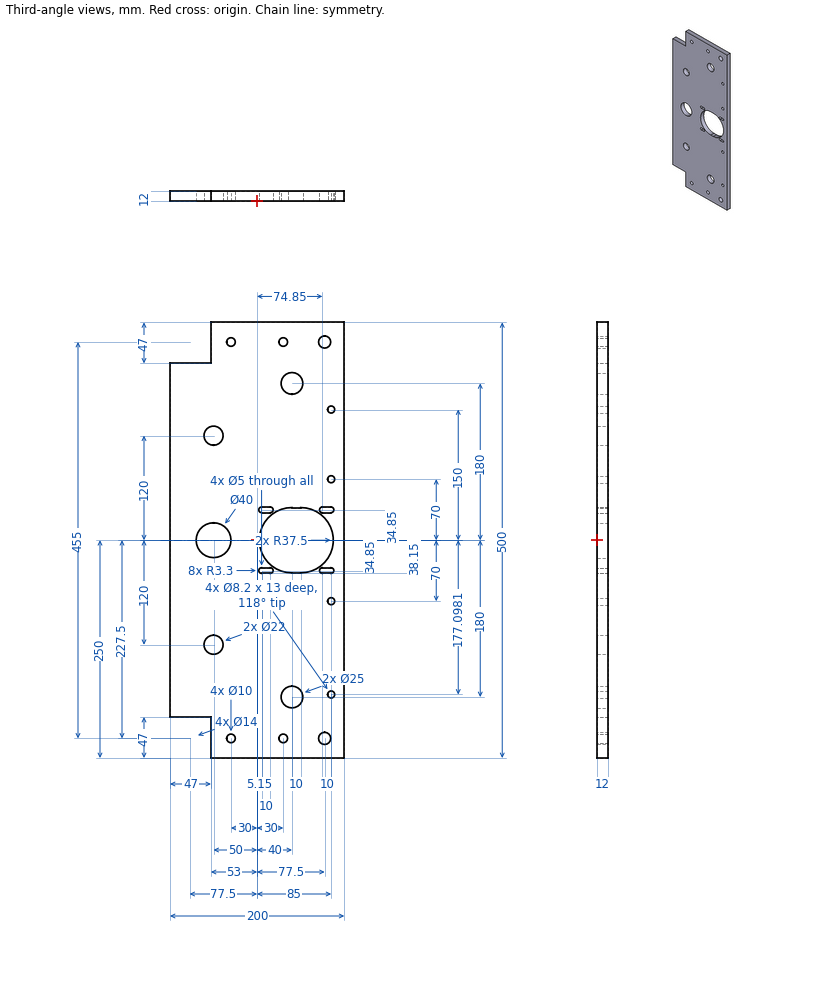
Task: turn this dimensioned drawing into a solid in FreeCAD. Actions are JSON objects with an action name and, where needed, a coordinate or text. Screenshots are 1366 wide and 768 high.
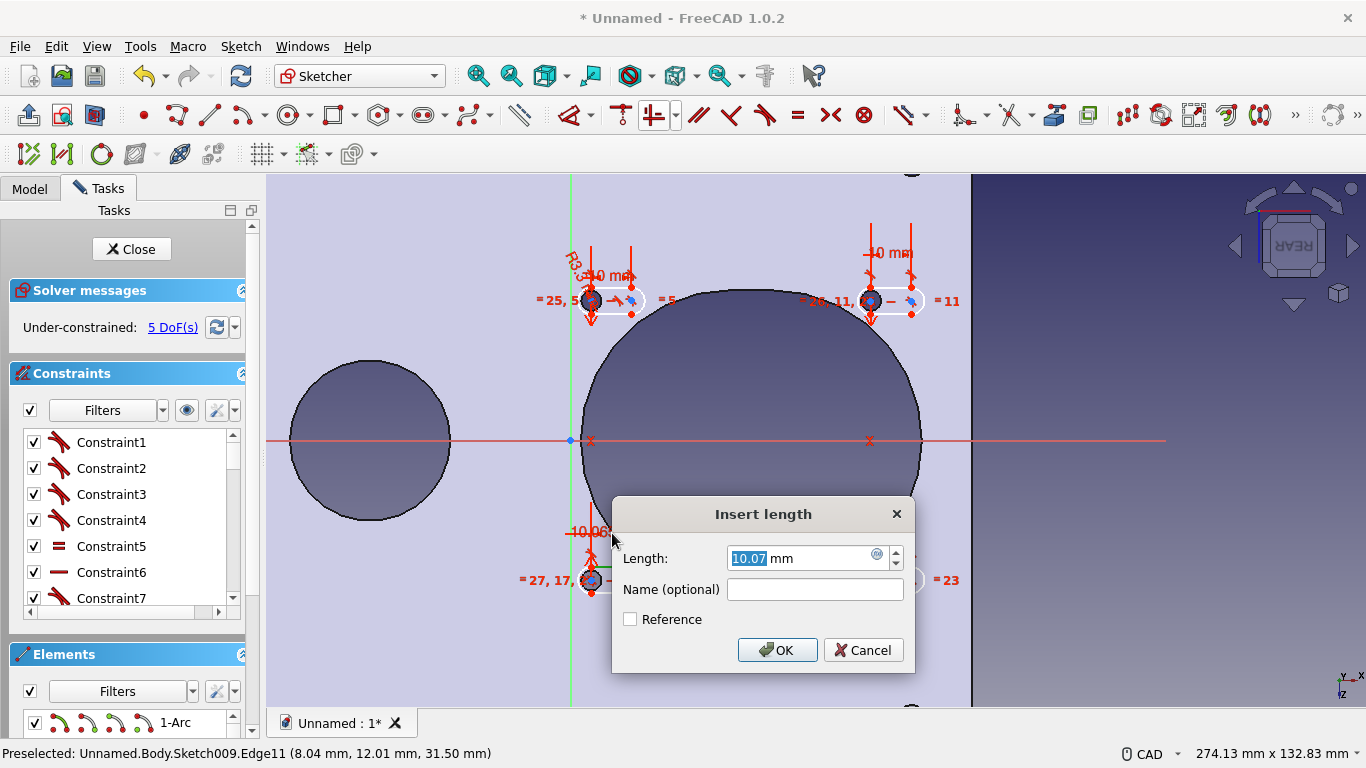
{"action": "type", "text": "10"}
{"action": "key", "text": "Return"}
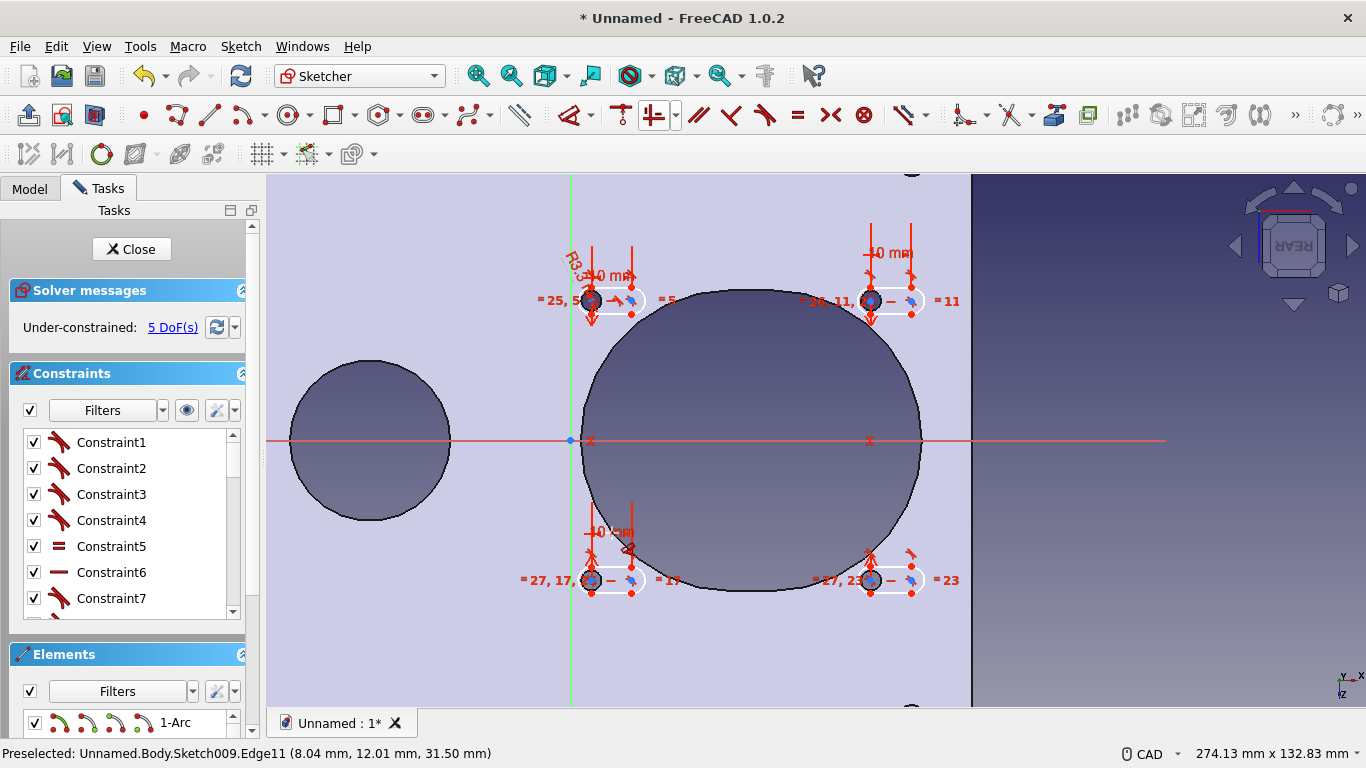
{"action": "left_click", "coordinate": [883, 567]}
{"action": "left_click", "coordinate": [891, 533]}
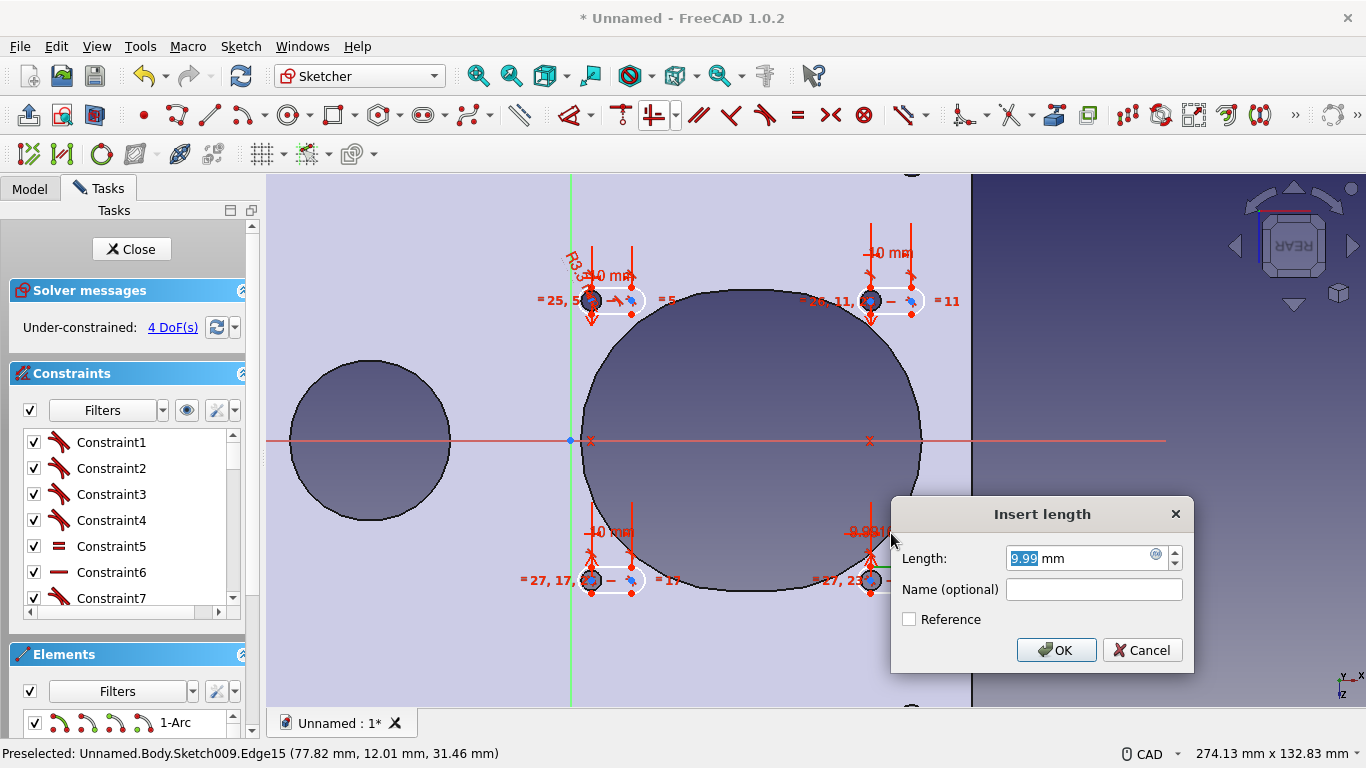
{"action": "type", "text": "10"}
{"action": "key", "text": "Return"}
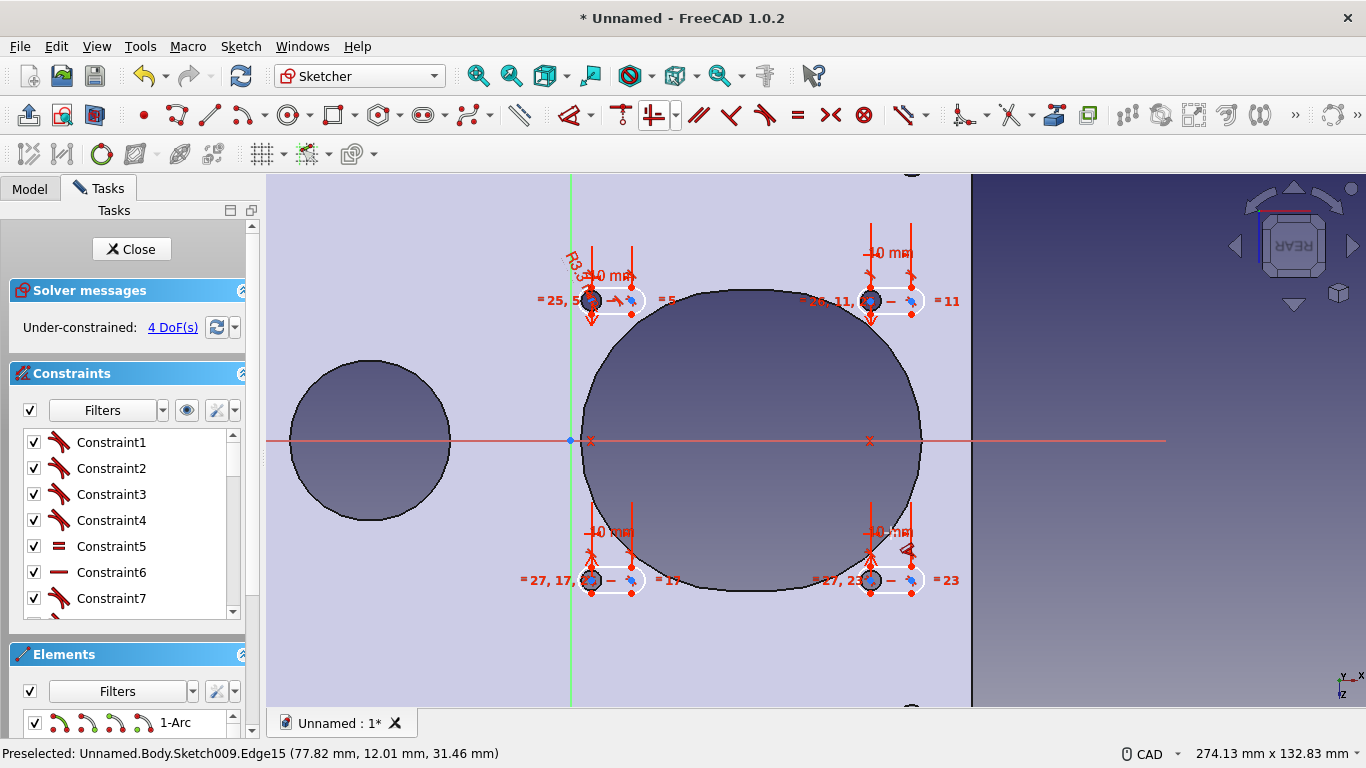
{"action": "scroll", "coordinate": [592, 288], "scroll_direction": "up", "scroll_amount": 4}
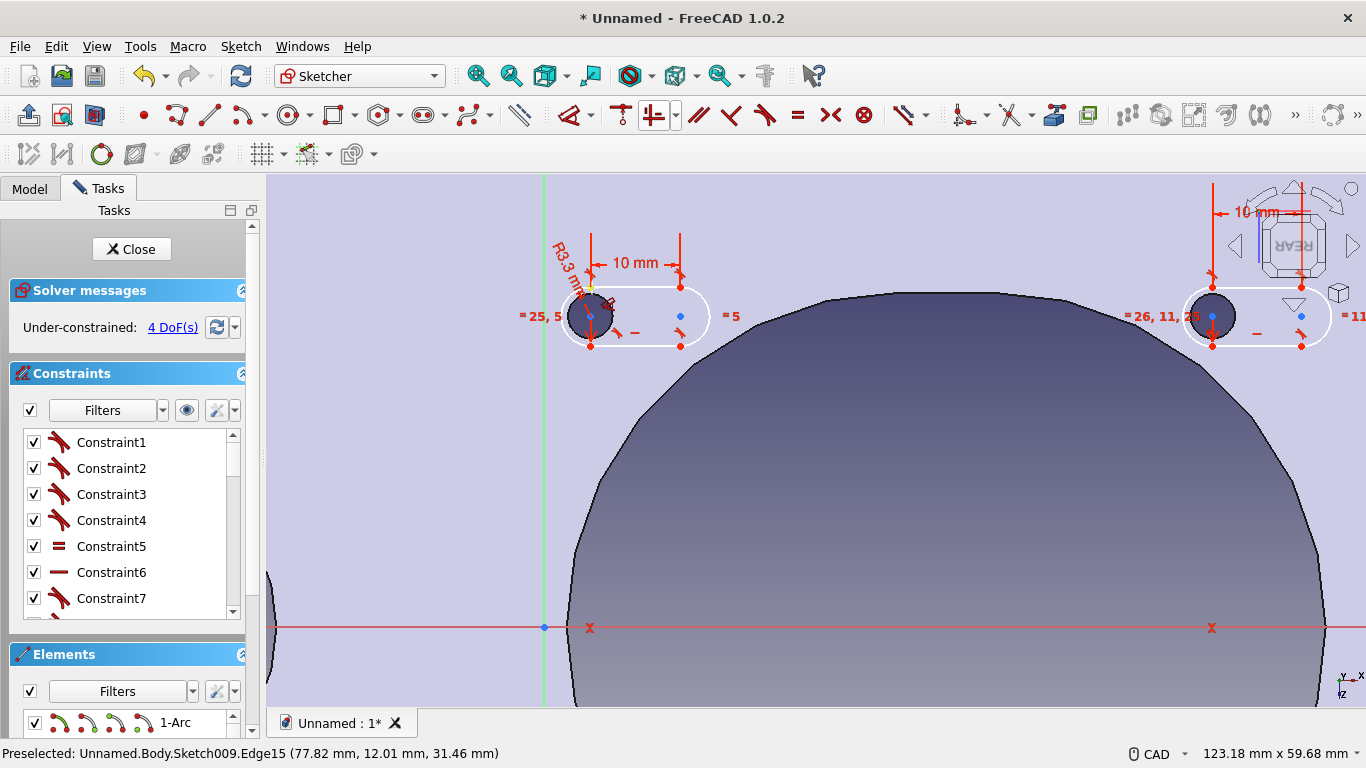
{"action": "left_click", "coordinate": [591, 287]}
{"action": "left_click", "coordinate": [568, 661]}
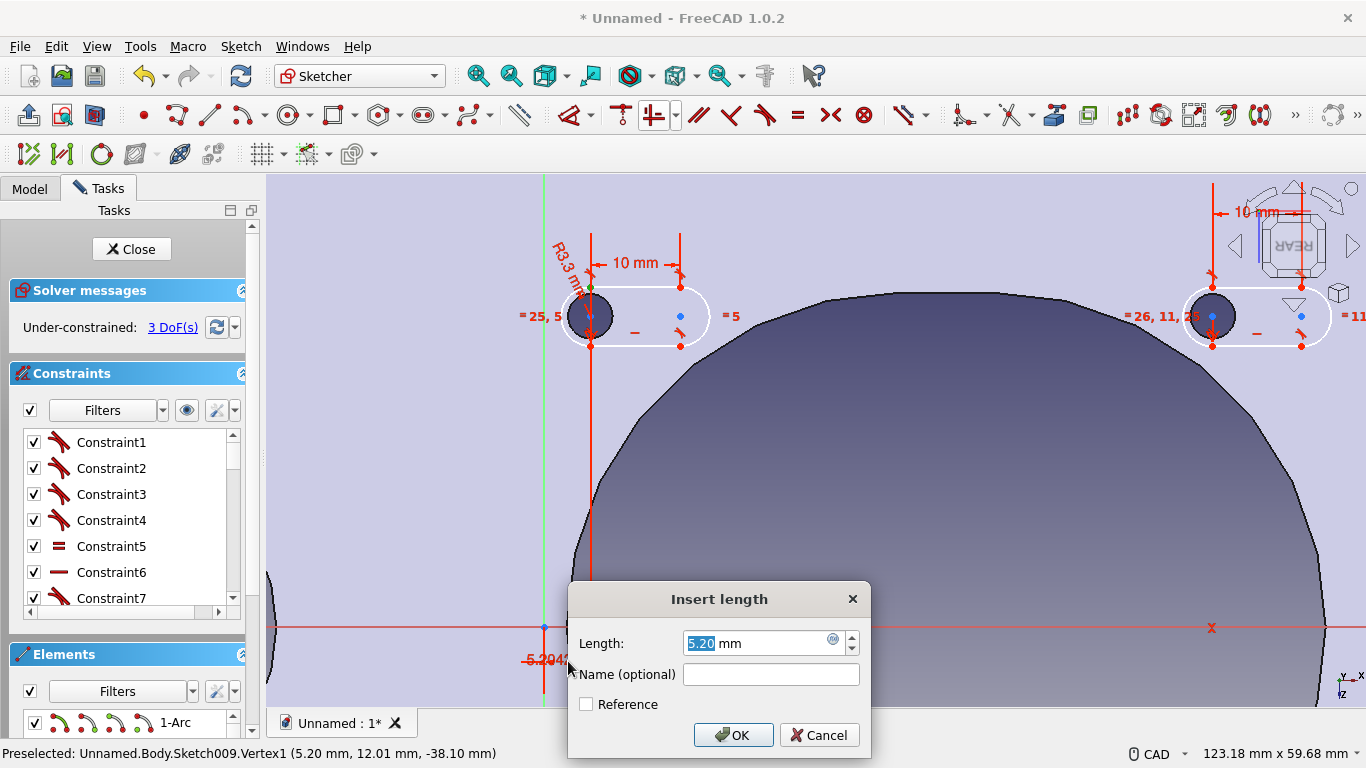
{"action": "type", "text": "5.15"}
{"action": "key", "text": "Return"}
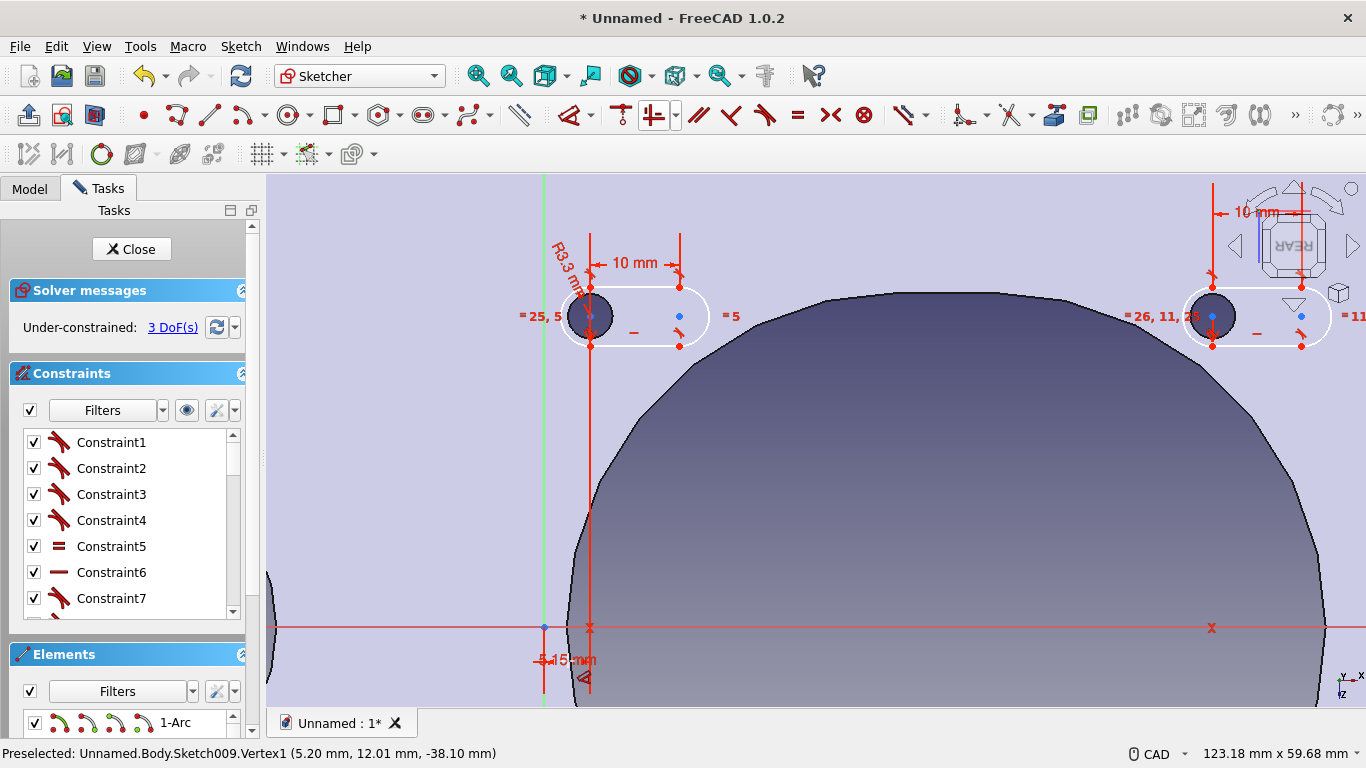
{"action": "left_click", "coordinate": [590, 287]}
{"action": "left_click", "coordinate": [510, 457]}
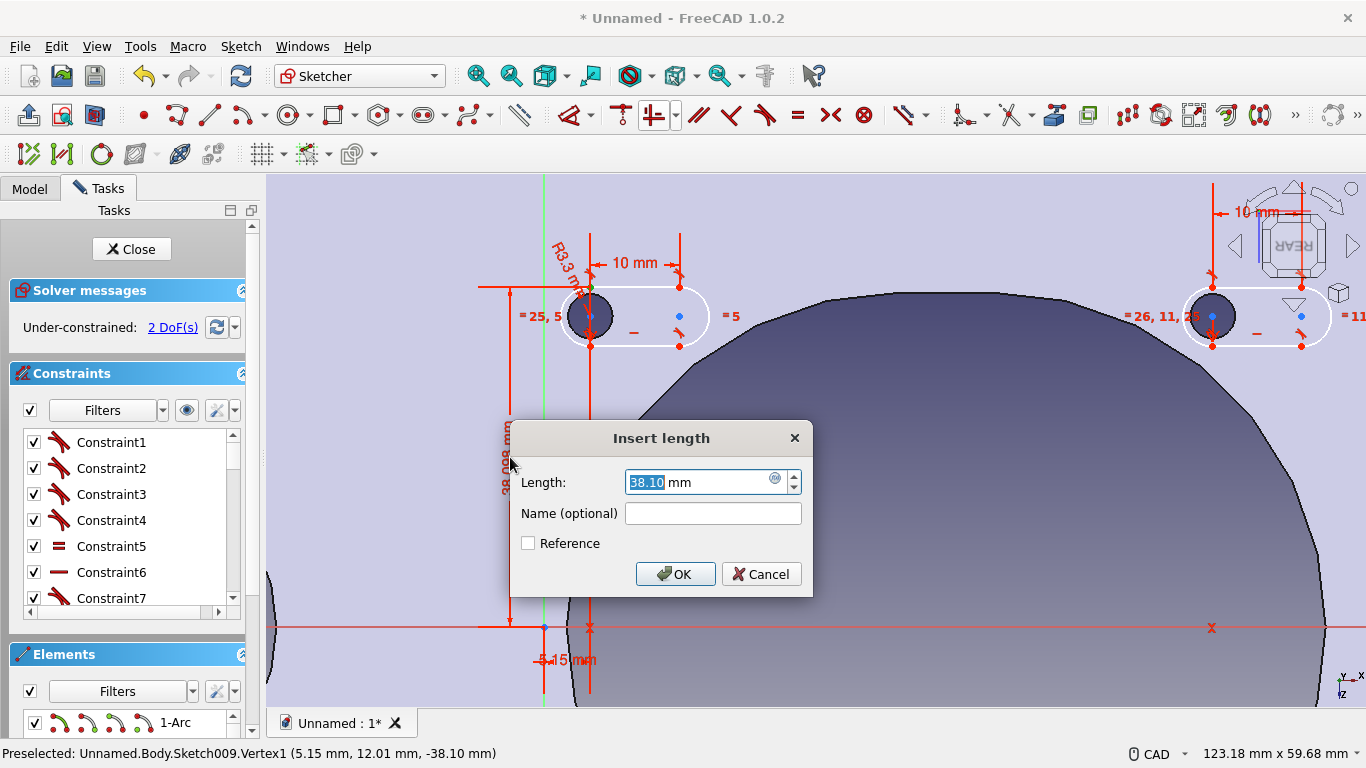
{"action": "type", "text": "38.15"}
{"action": "key", "text": "Return"}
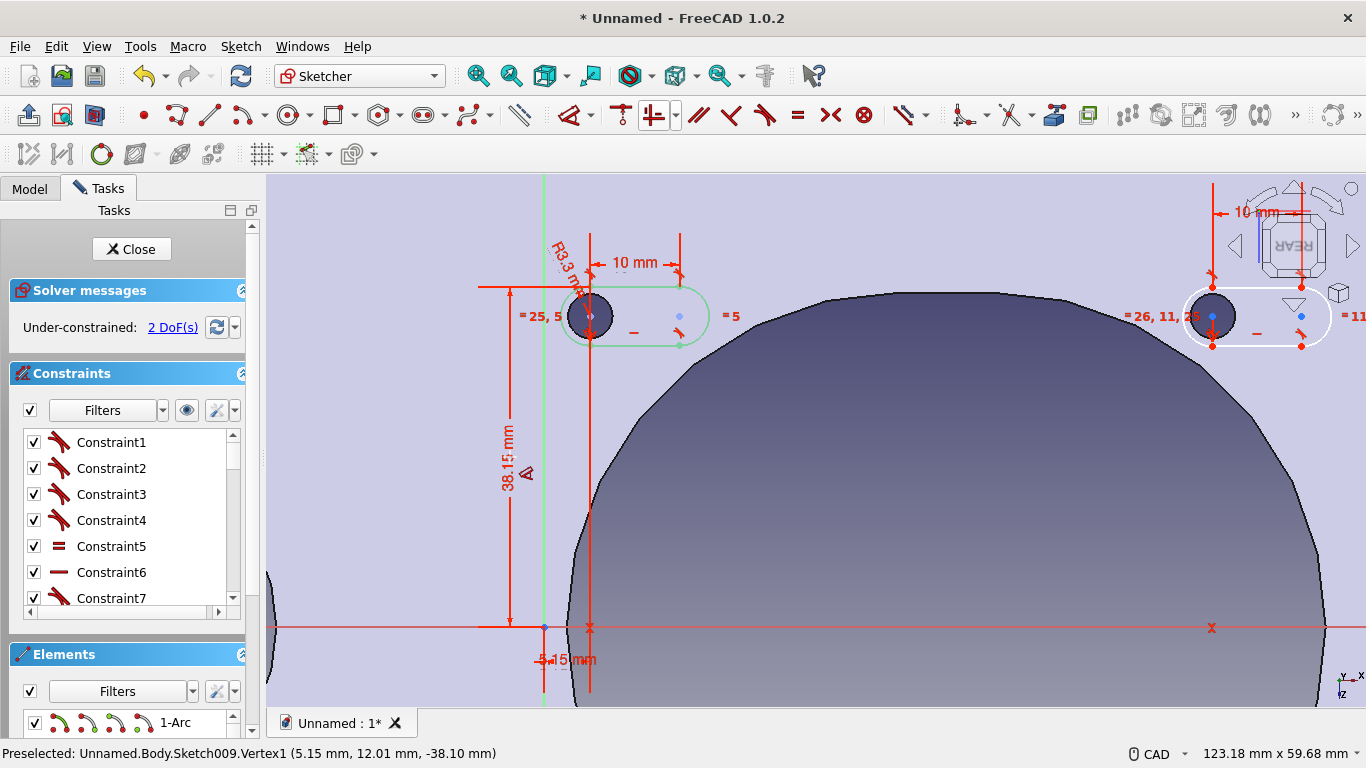
{"action": "scroll", "coordinate": [592, 288], "scroll_direction": "down", "scroll_amount": 4}